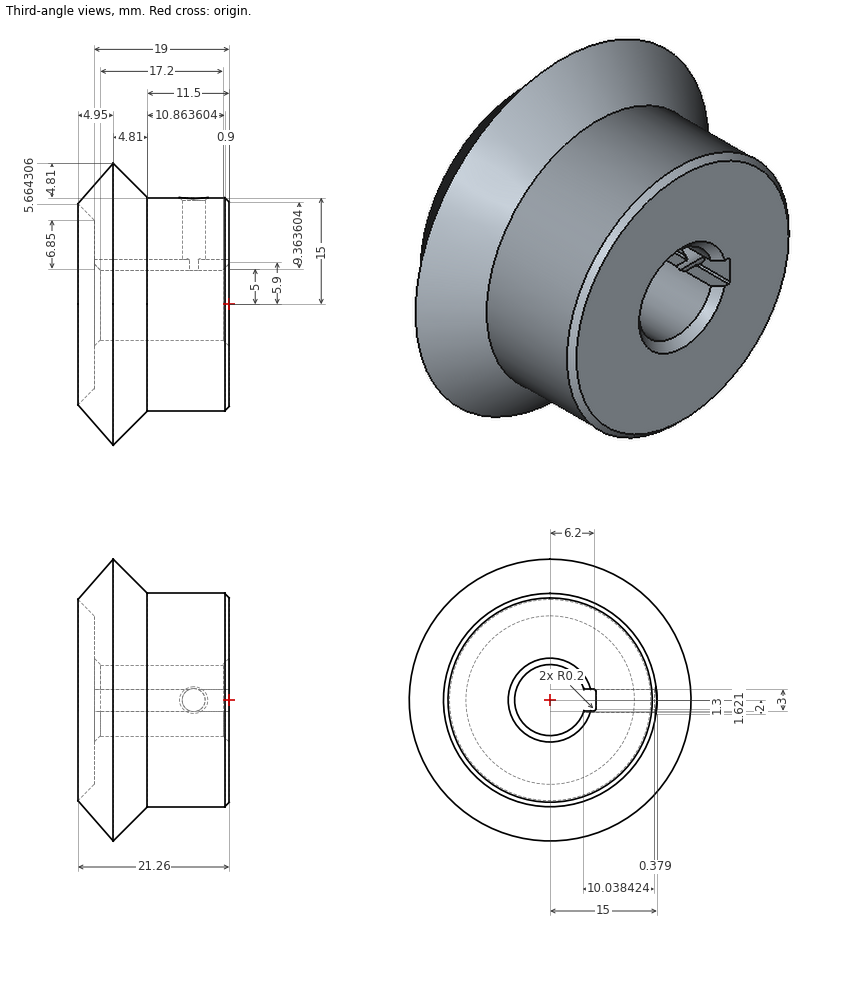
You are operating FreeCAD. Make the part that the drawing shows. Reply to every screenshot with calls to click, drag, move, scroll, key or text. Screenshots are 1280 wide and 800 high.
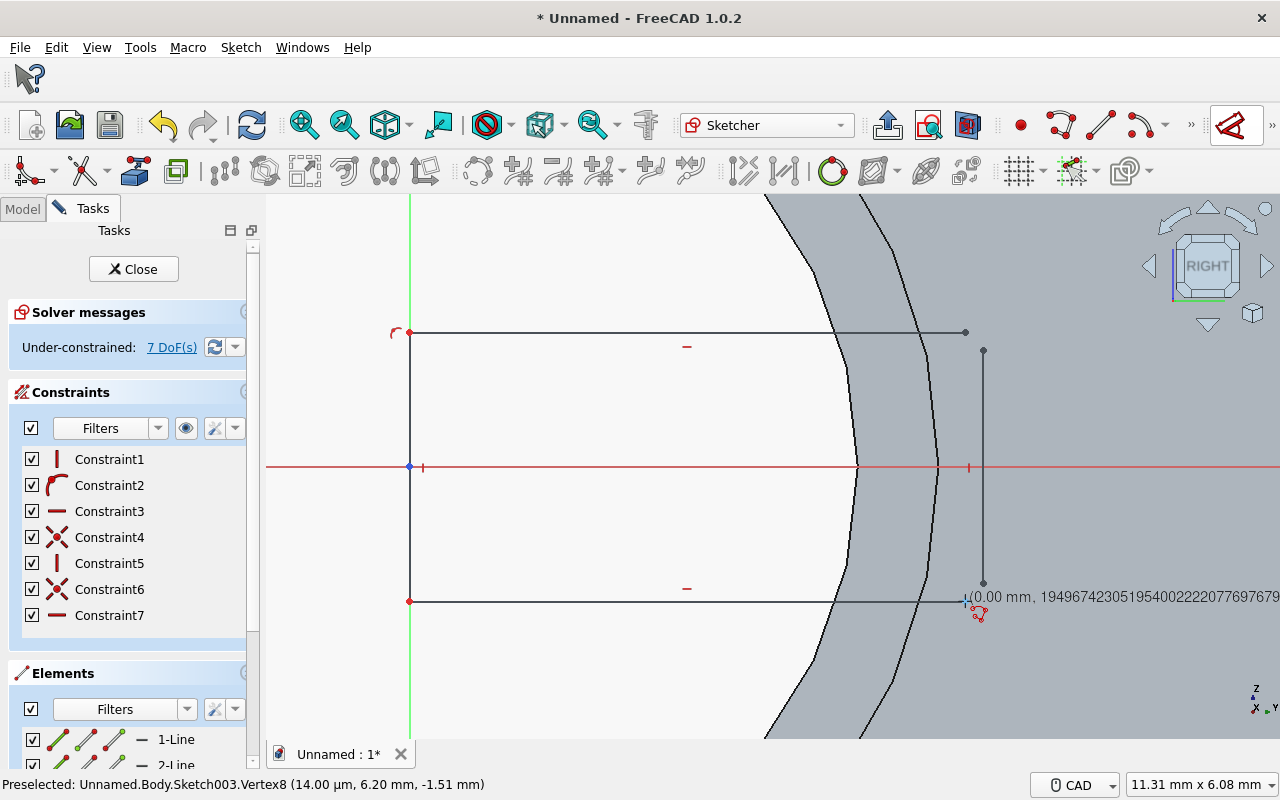
click(1168, 126)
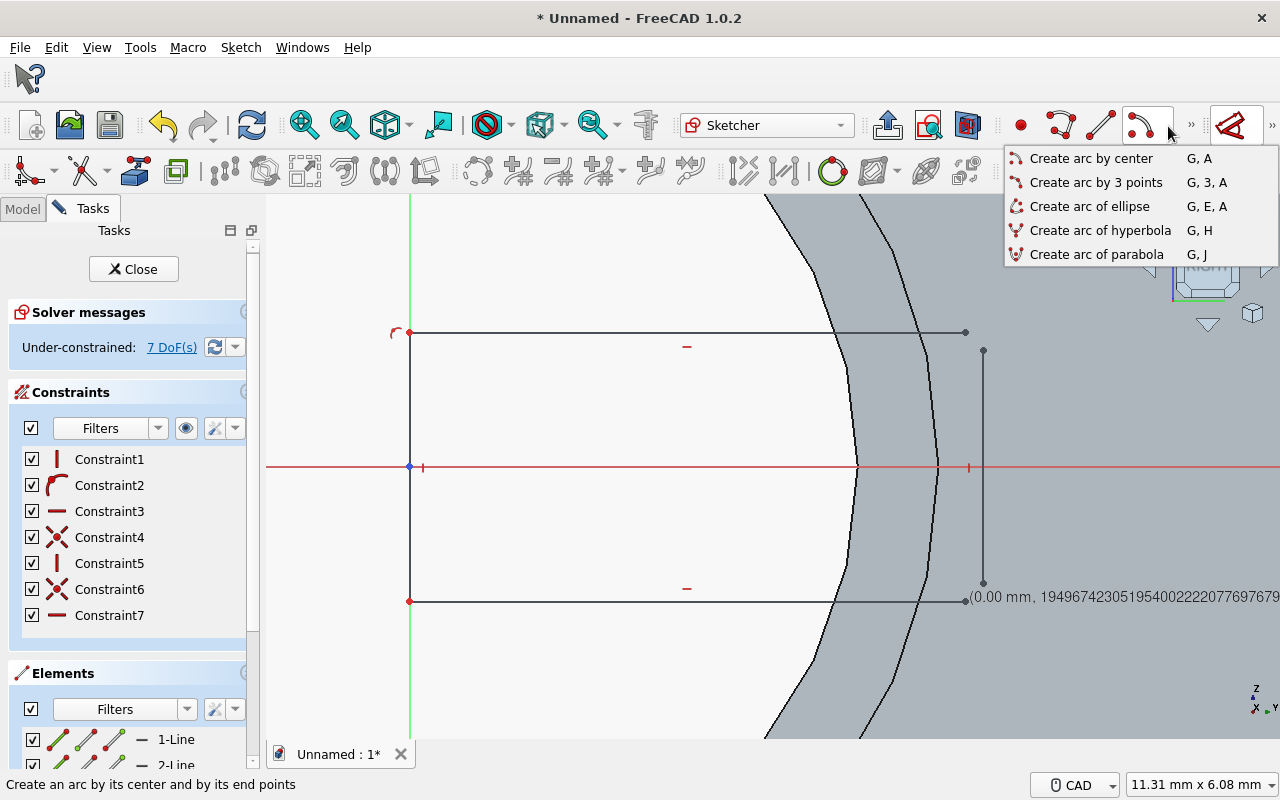
click(1142, 182)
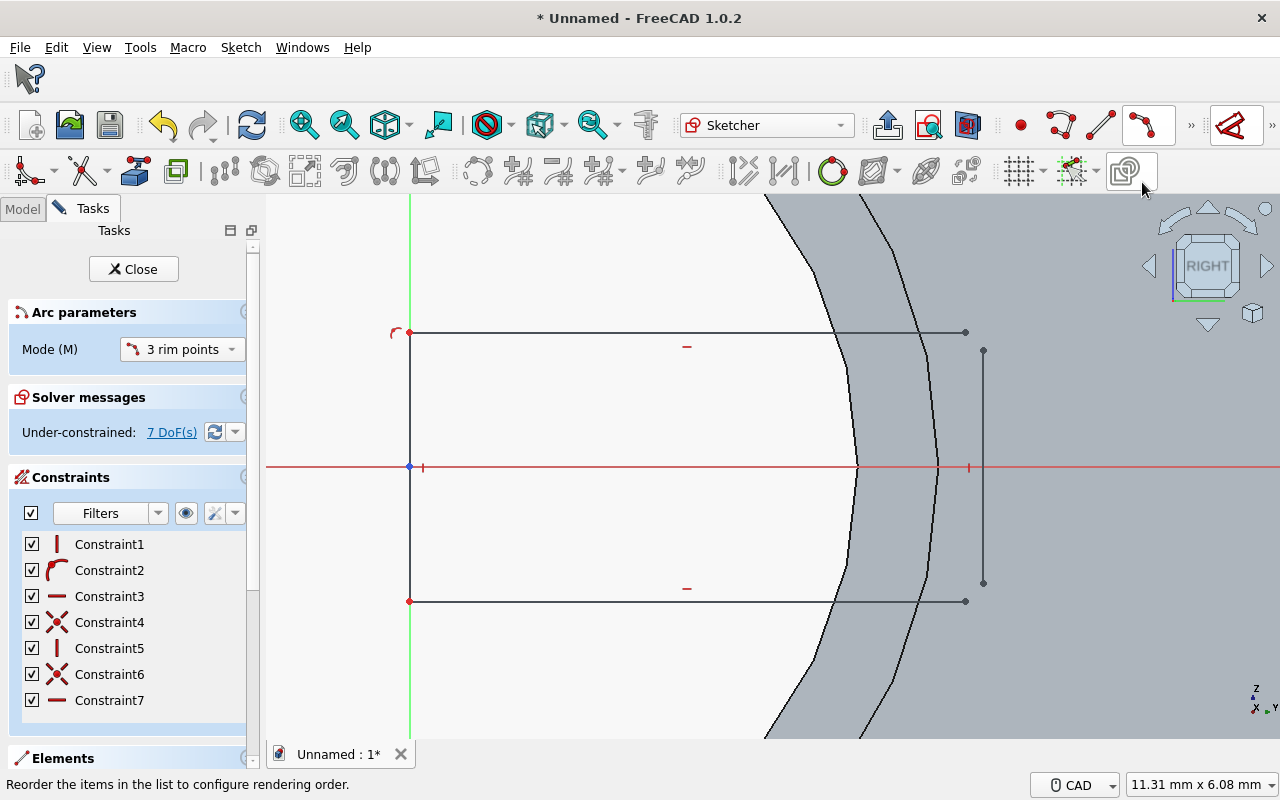
click(983, 351)
click(965, 333)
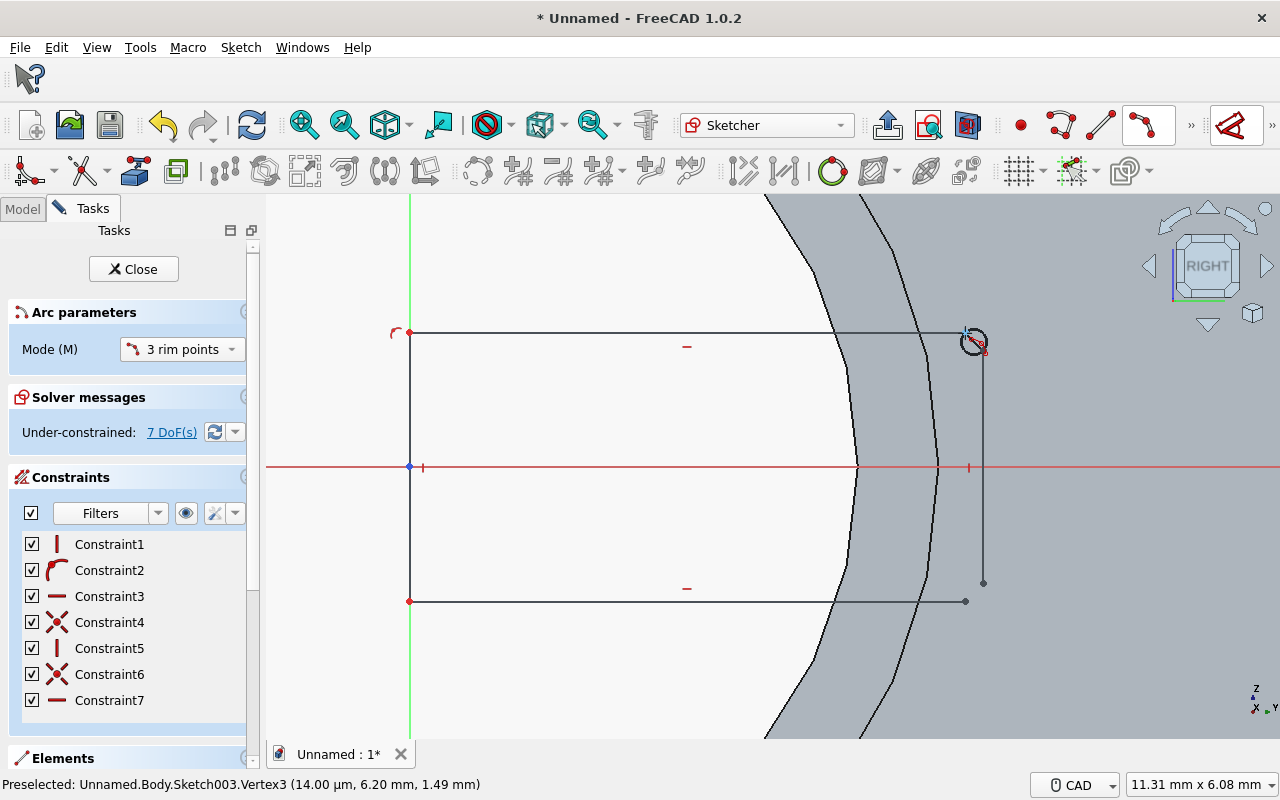
scroll(978, 337, up, 6)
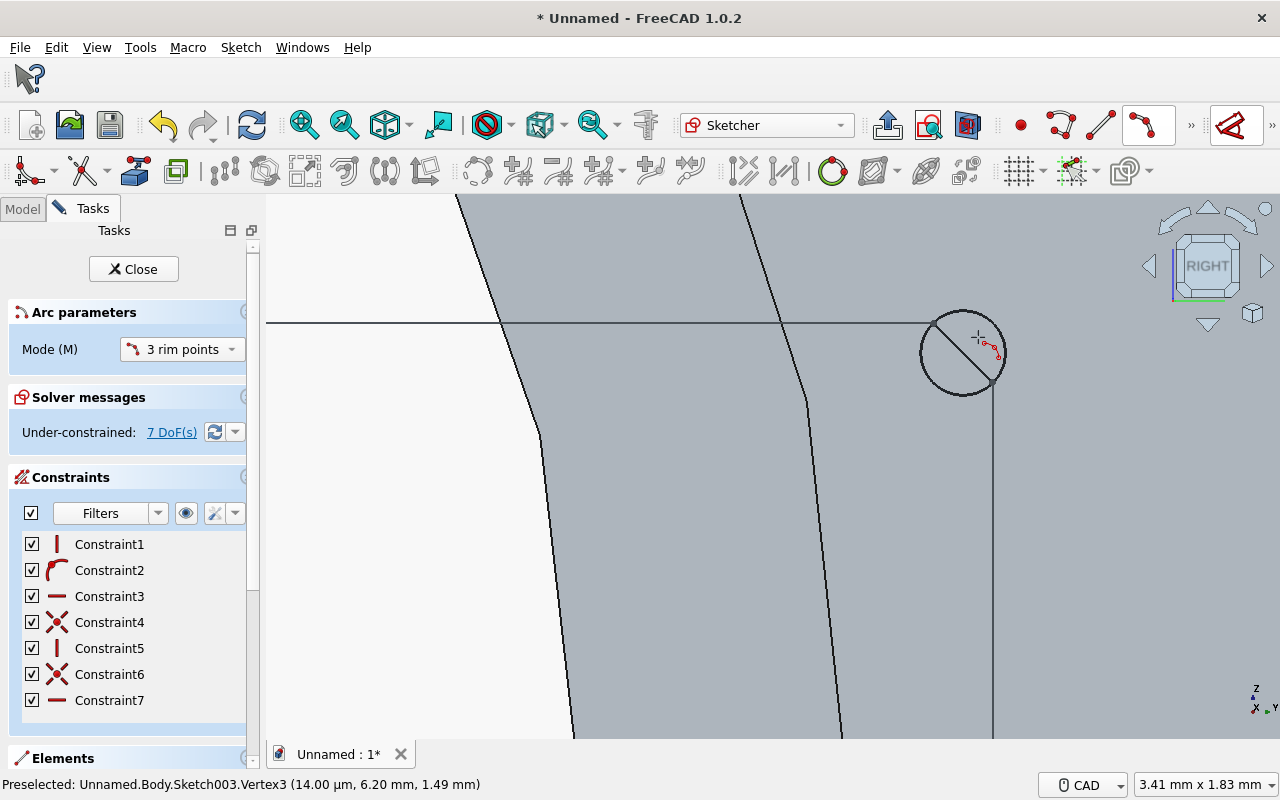
click(976, 337)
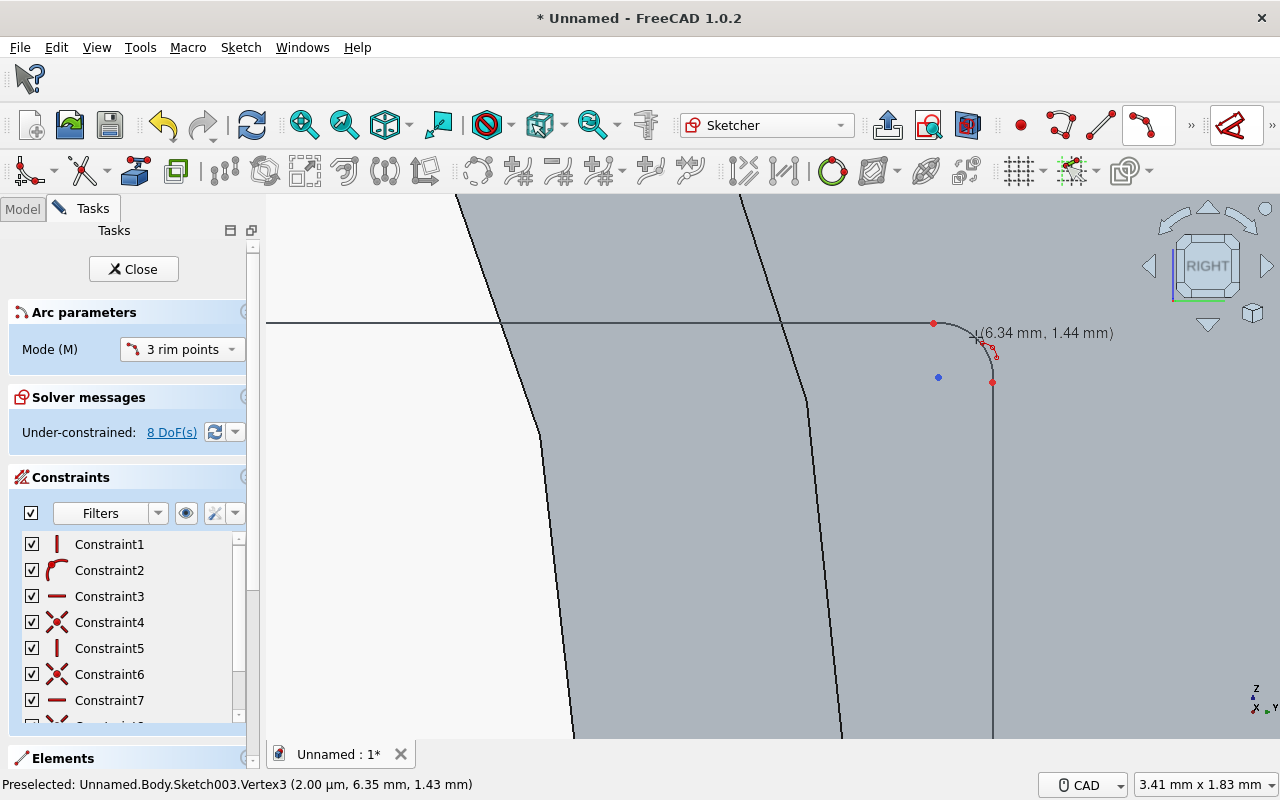
scroll(990, 337, down, 6)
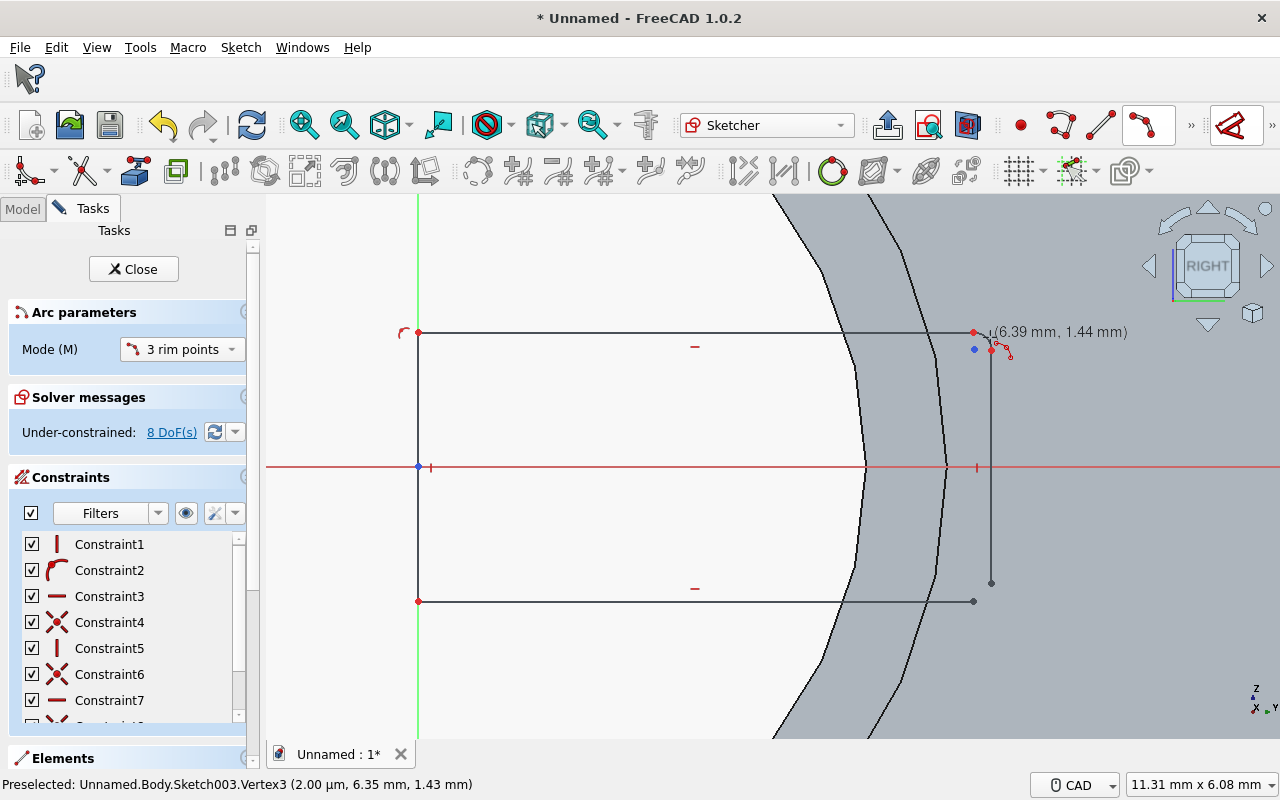
click(973, 602)
click(991, 584)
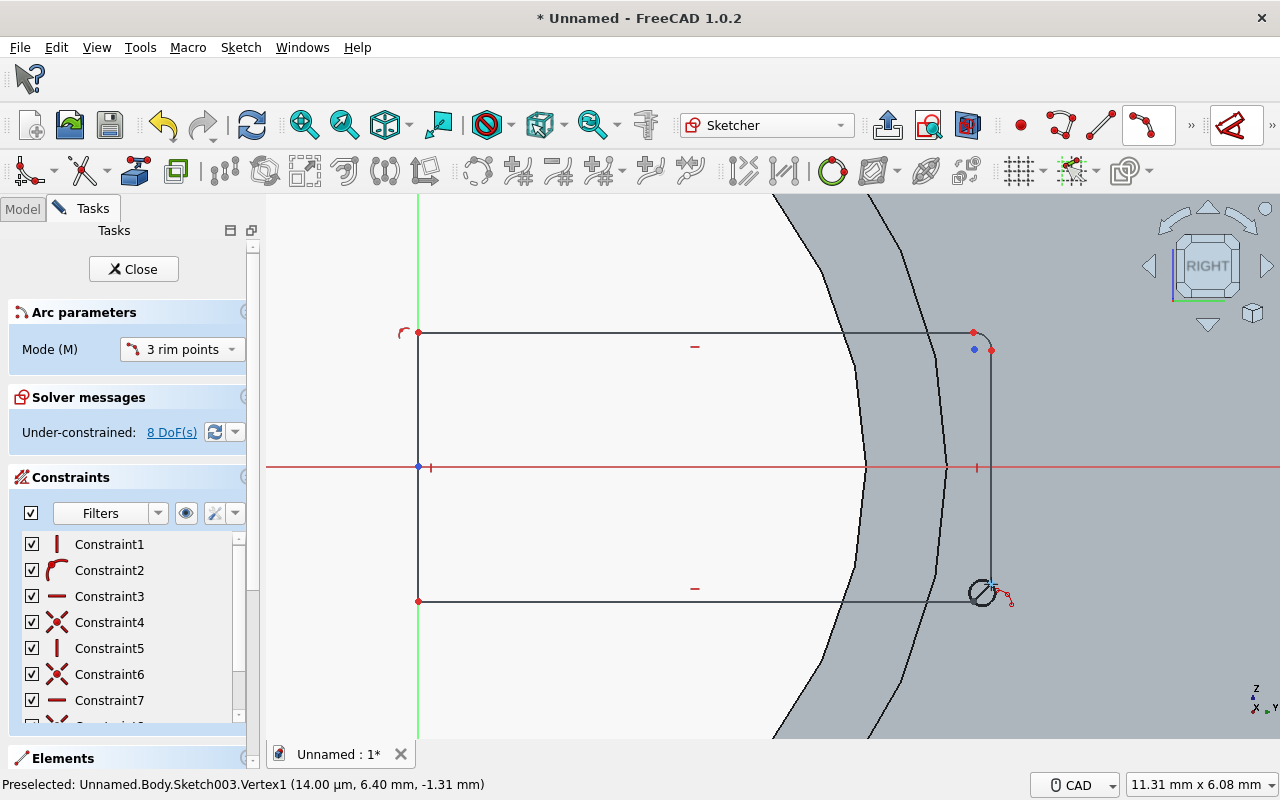
scroll(986, 596, up, 6)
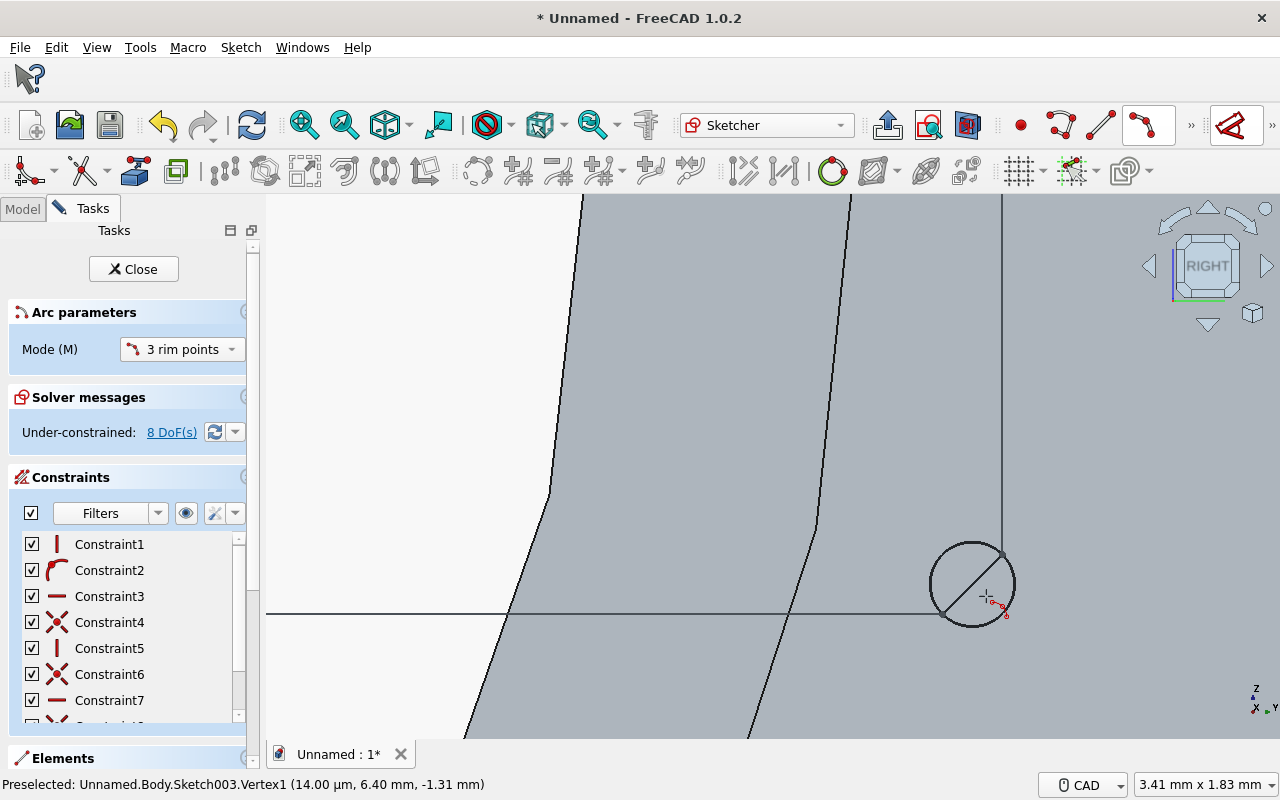
click(986, 593)
key(Escape)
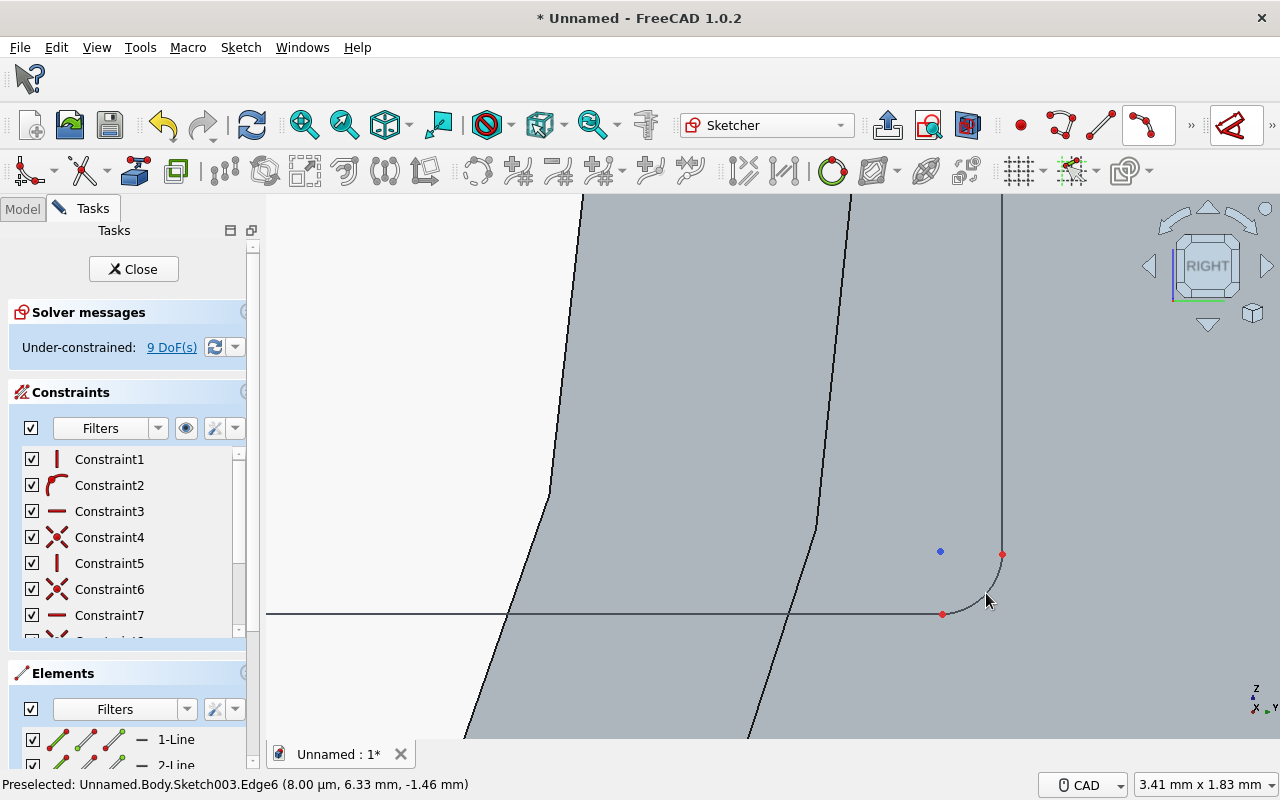
click(1002, 322)